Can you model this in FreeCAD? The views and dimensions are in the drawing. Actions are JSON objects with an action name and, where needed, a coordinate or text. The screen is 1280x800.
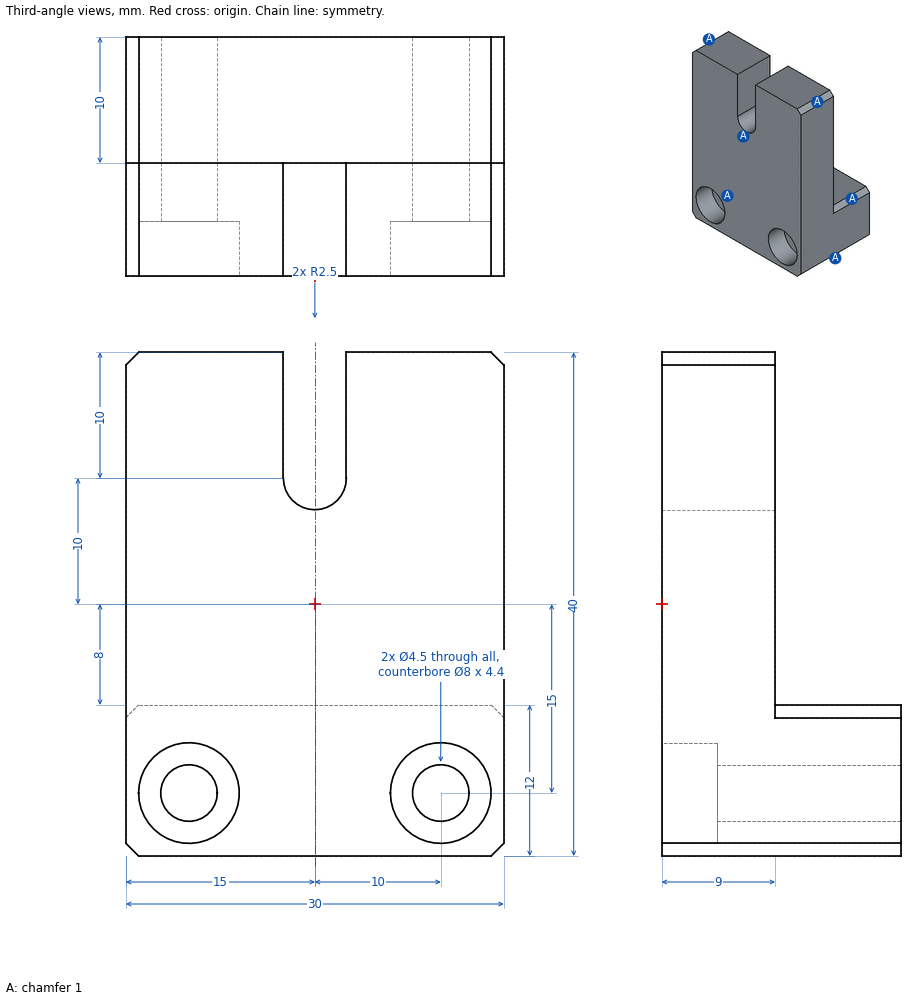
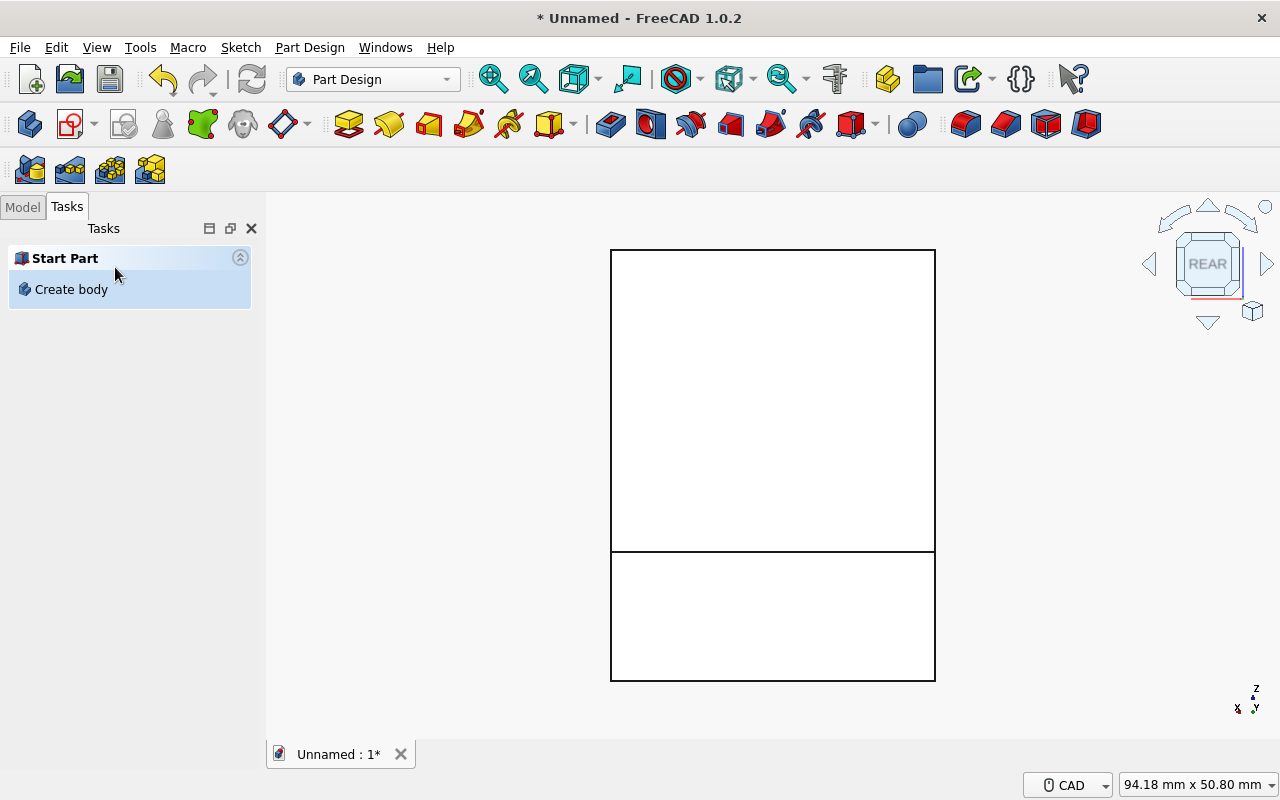
{"action": "key", "text": "0"}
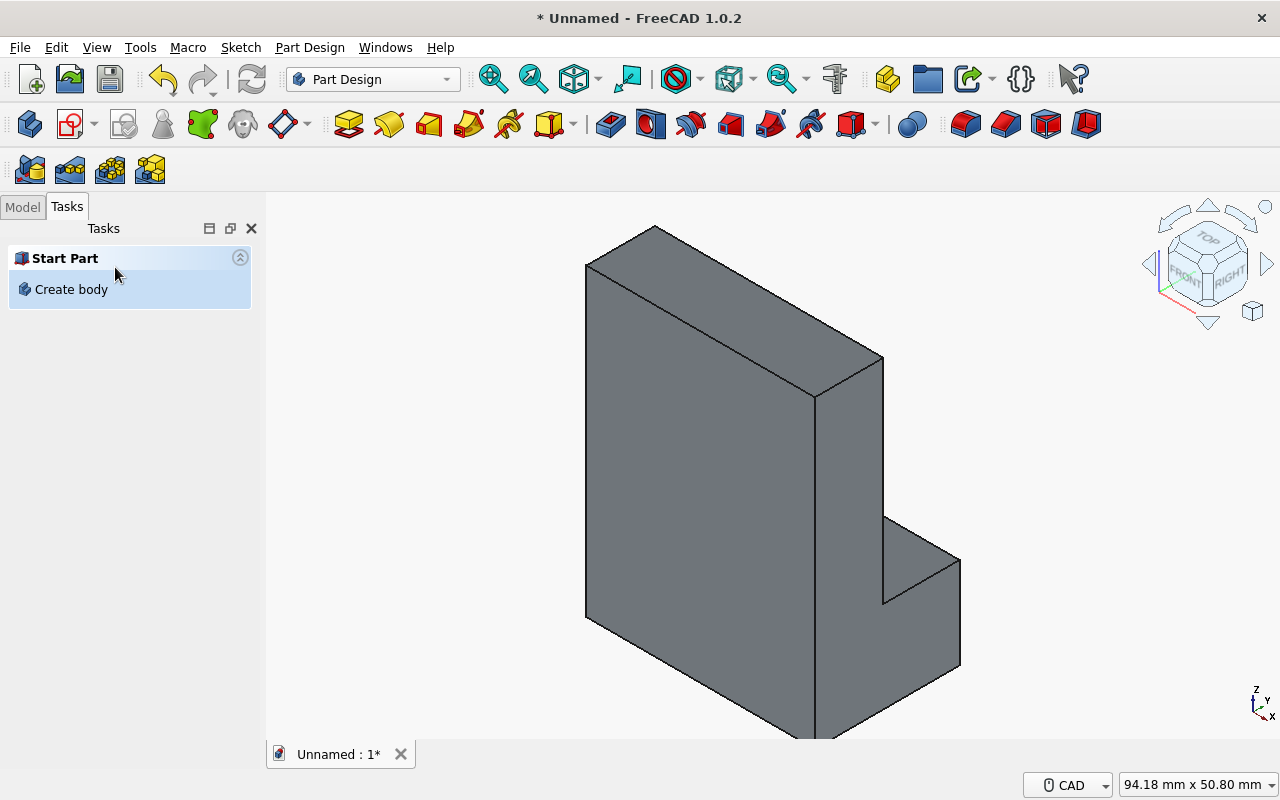
{"action": "key", "text": "v f"}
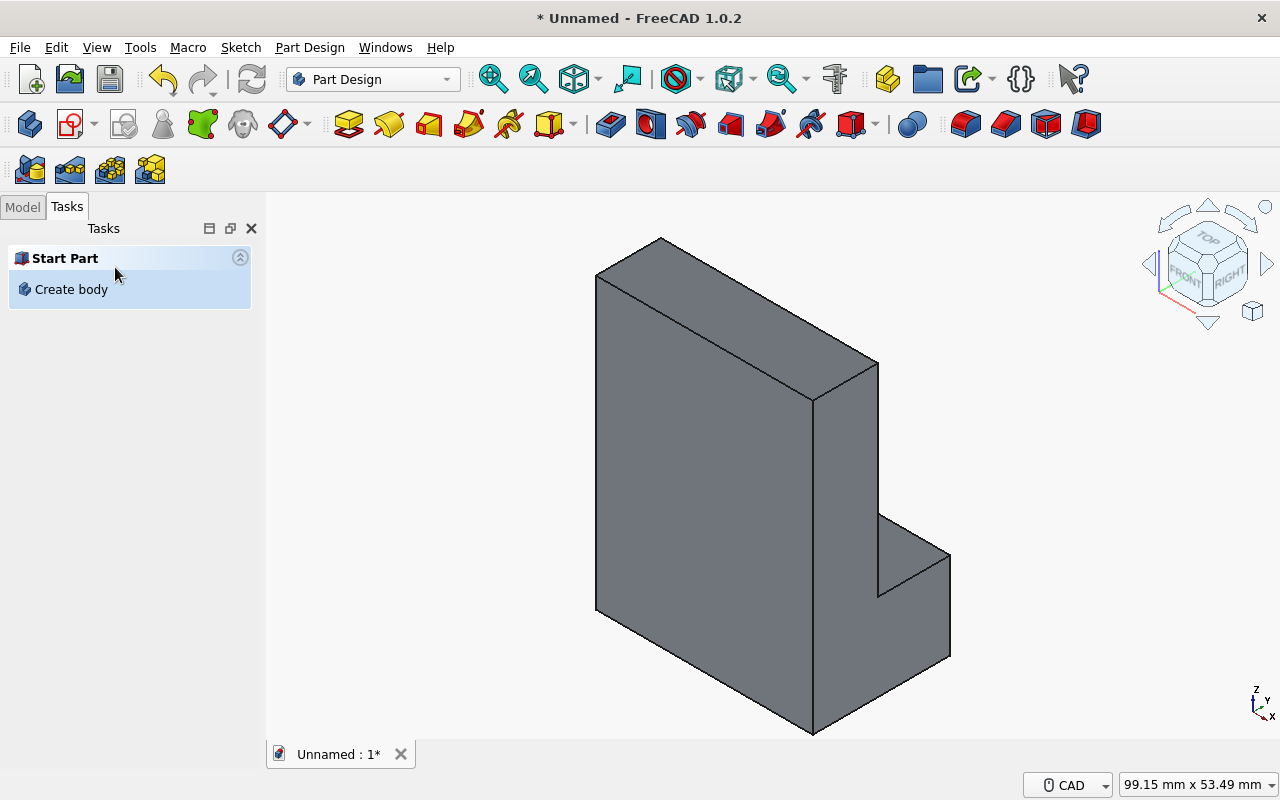
{"action": "left_click", "coordinate": [704, 504]}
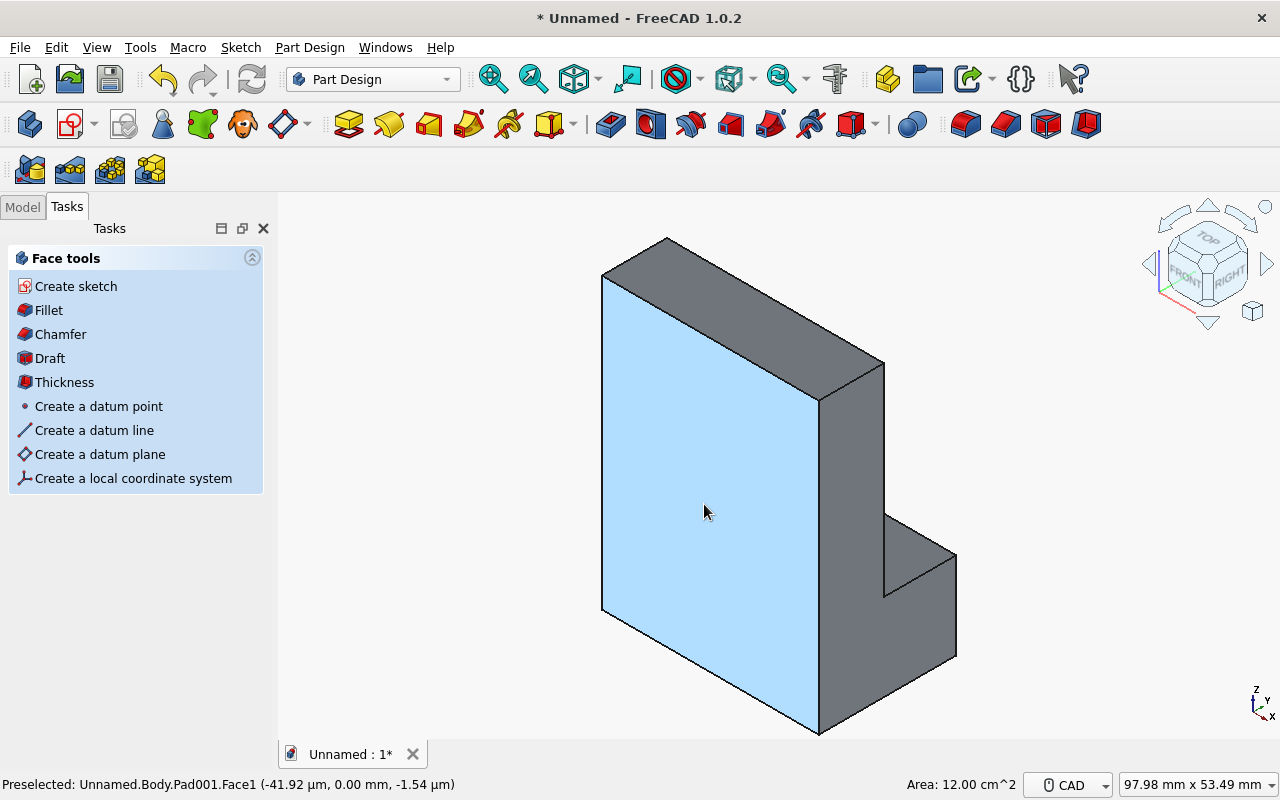
{"action": "left_click", "coordinate": [70, 124]}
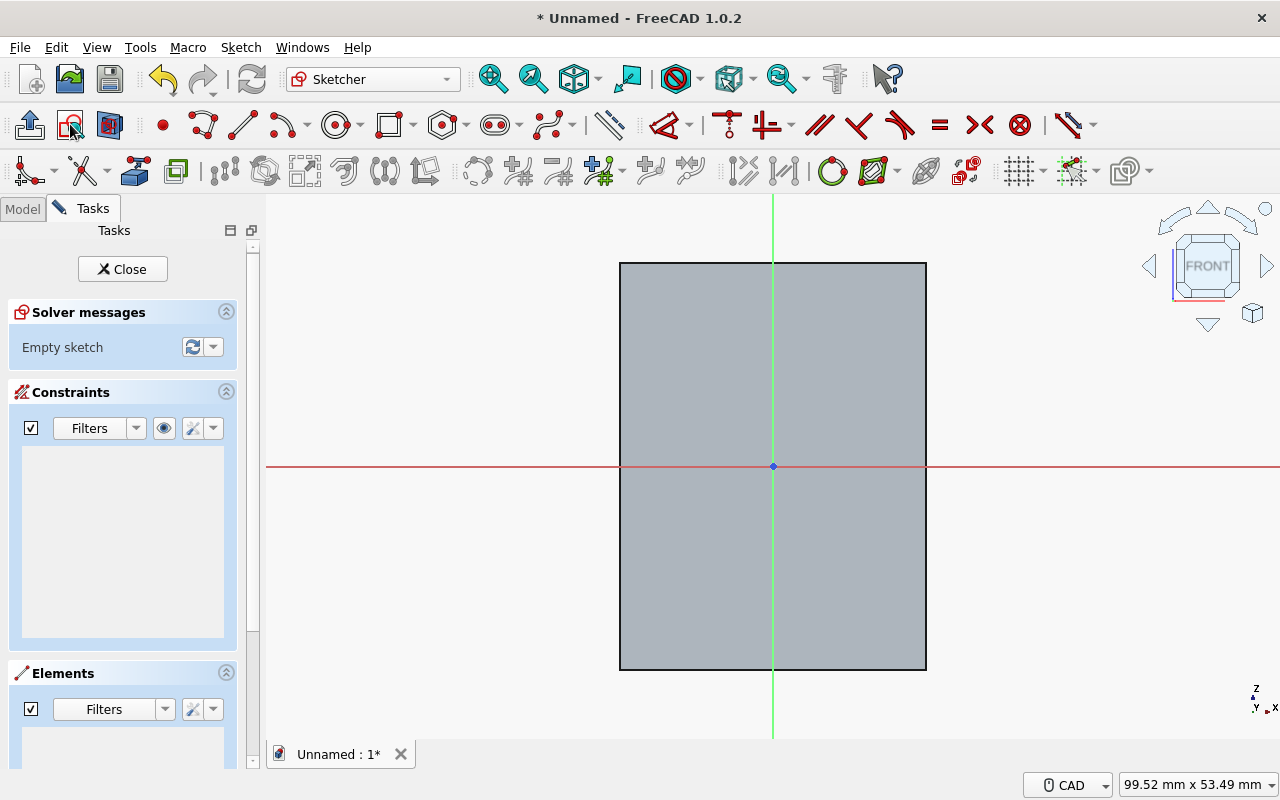
{"action": "scroll", "coordinate": [856, 661], "scroll_direction": "up", "scroll_amount": 3}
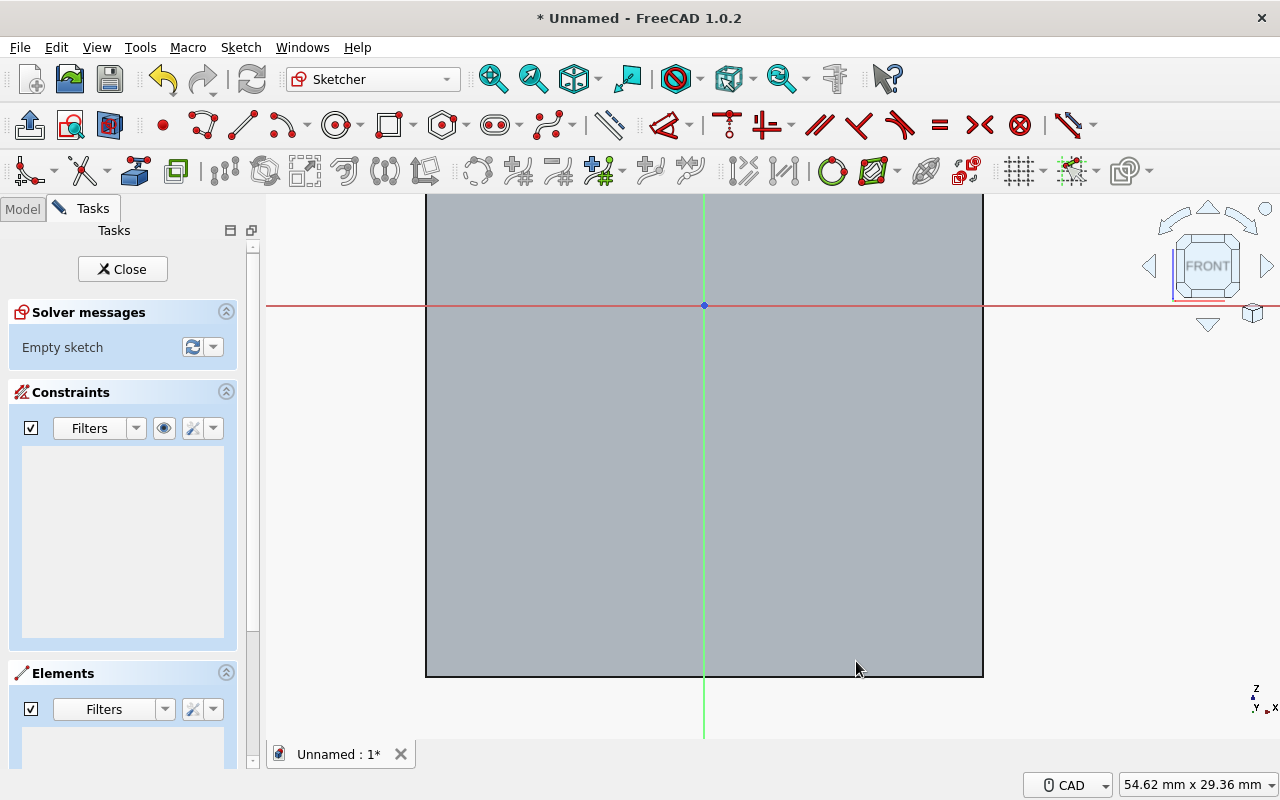
{"action": "key", "text": "g c"}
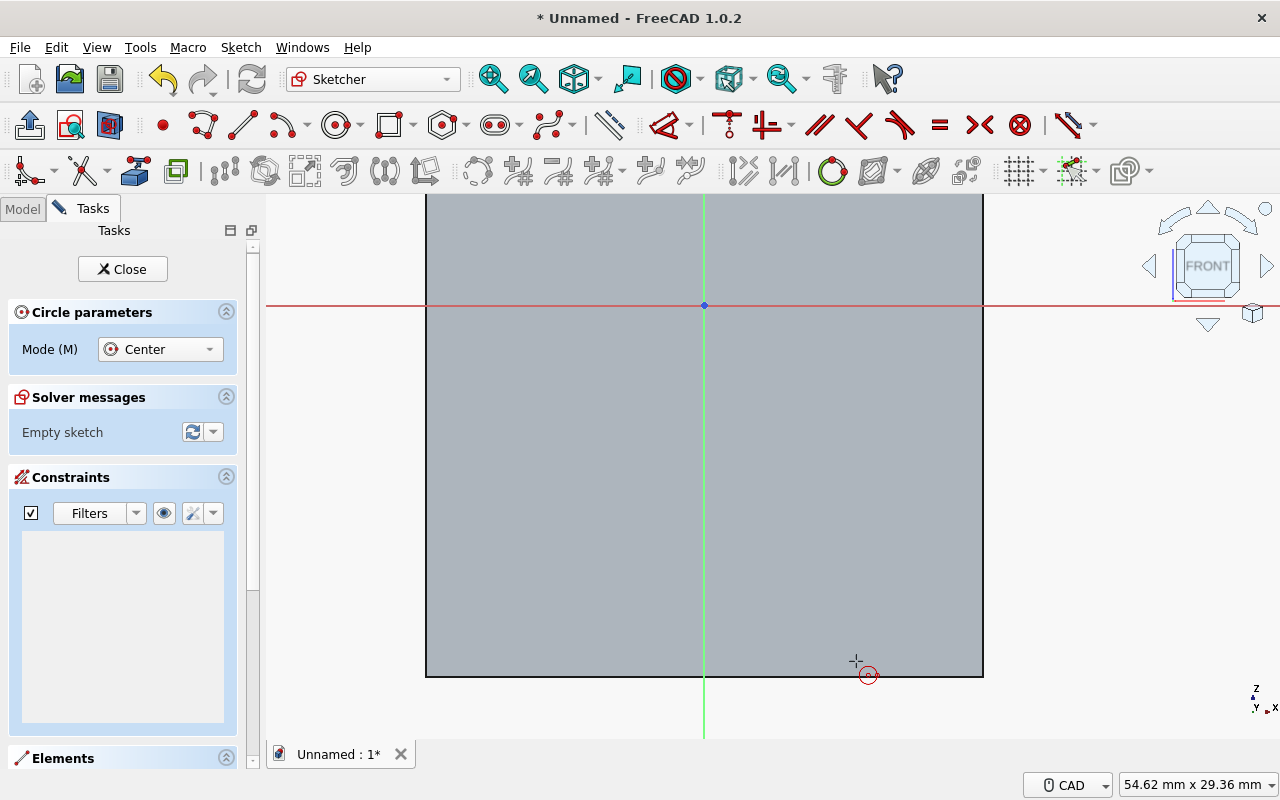
{"action": "left_click", "coordinate": [890, 584]}
{"action": "mouse_move", "coordinate": [919, 555]}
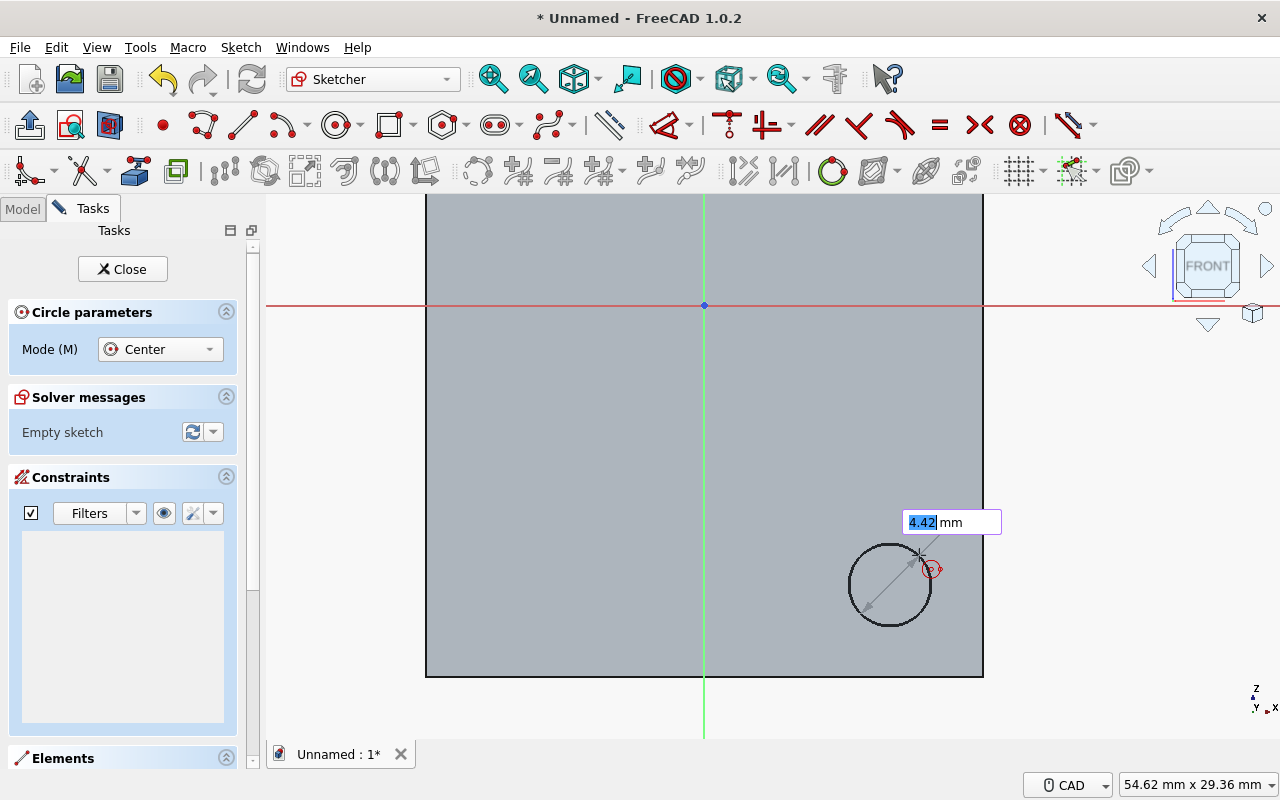
{"action": "type", "text": "4.5"}
{"action": "key", "text": "Return"}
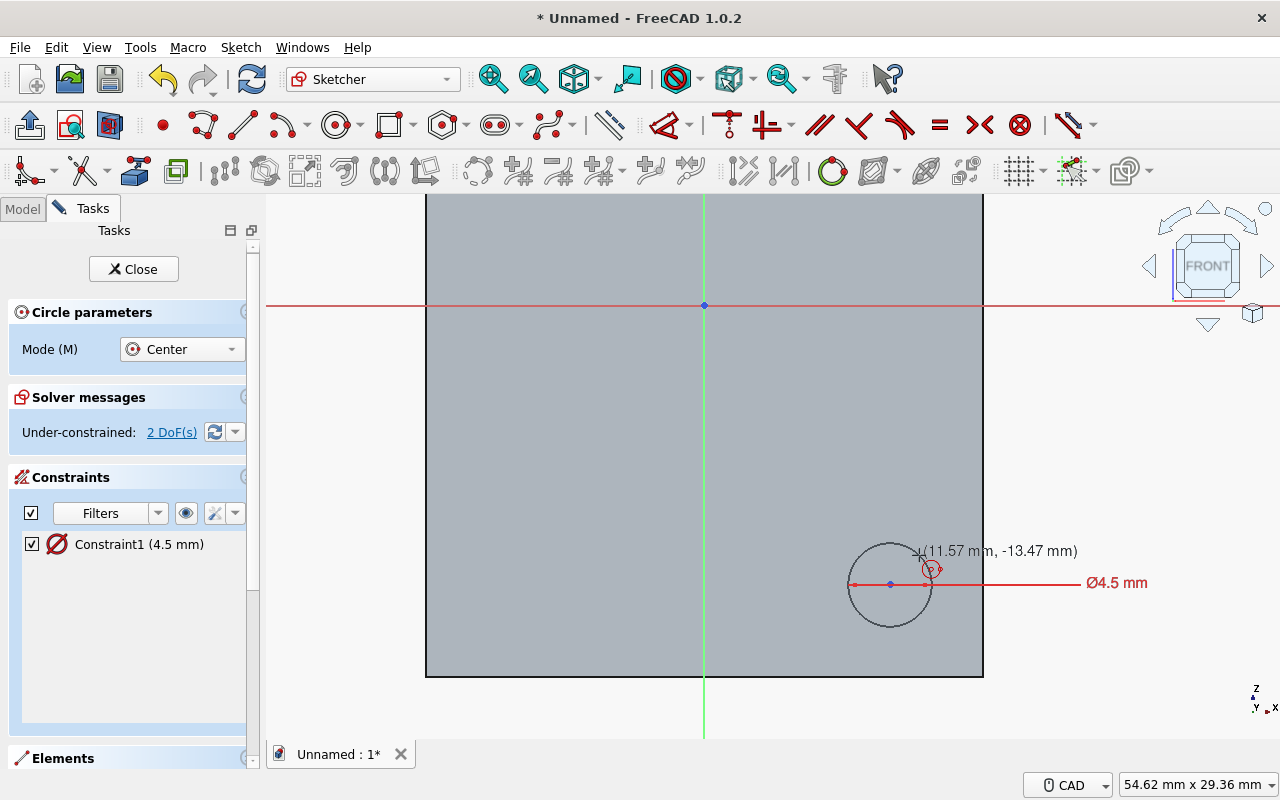
{"action": "left_click", "coordinate": [519, 584]}
{"action": "mouse_move", "coordinate": [548, 555]}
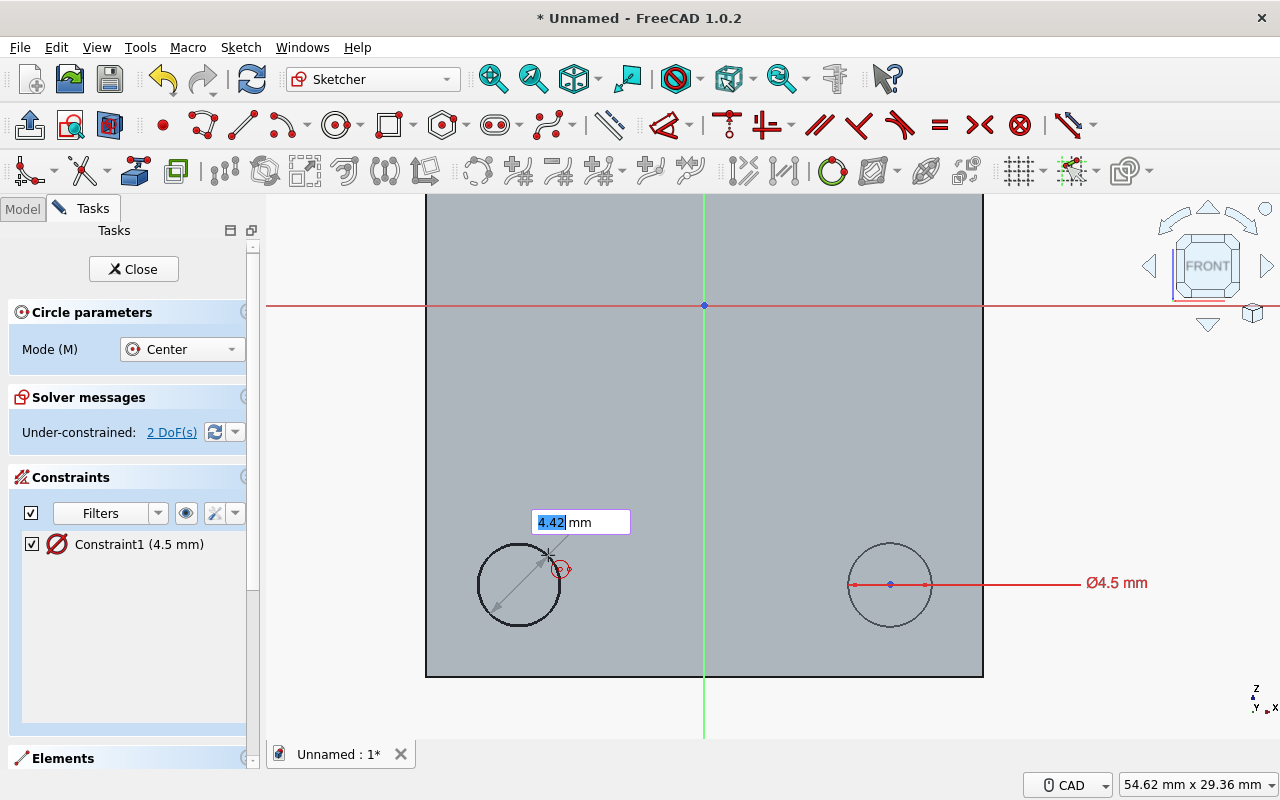
{"action": "type", "text": "4.5"}
{"action": "key", "text": "Return"}
{"action": "key", "text": "Escape"}